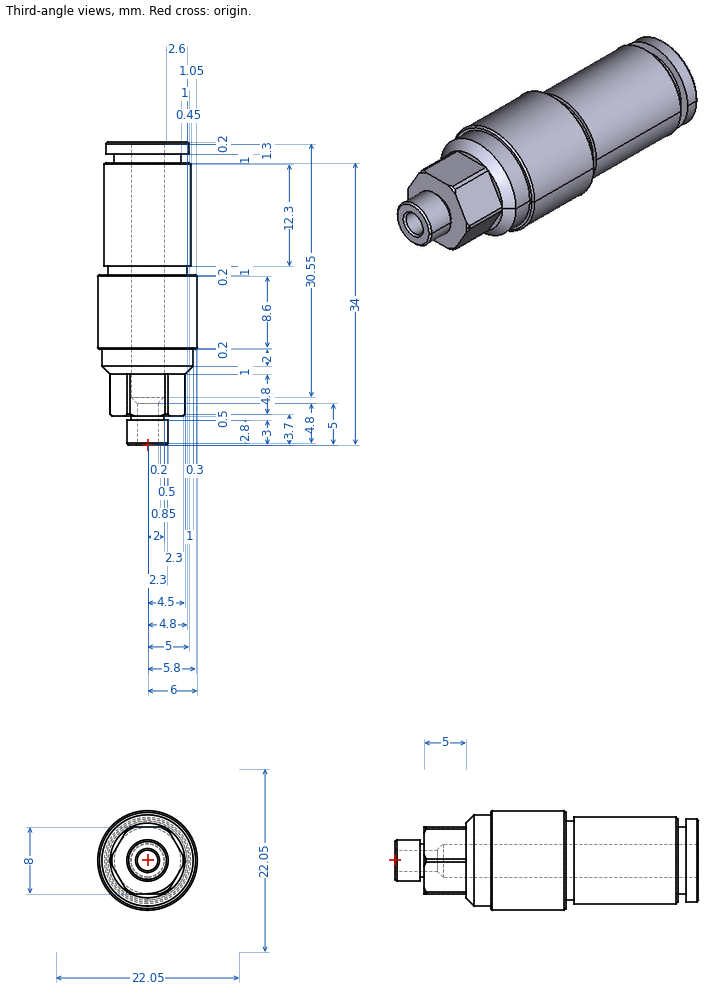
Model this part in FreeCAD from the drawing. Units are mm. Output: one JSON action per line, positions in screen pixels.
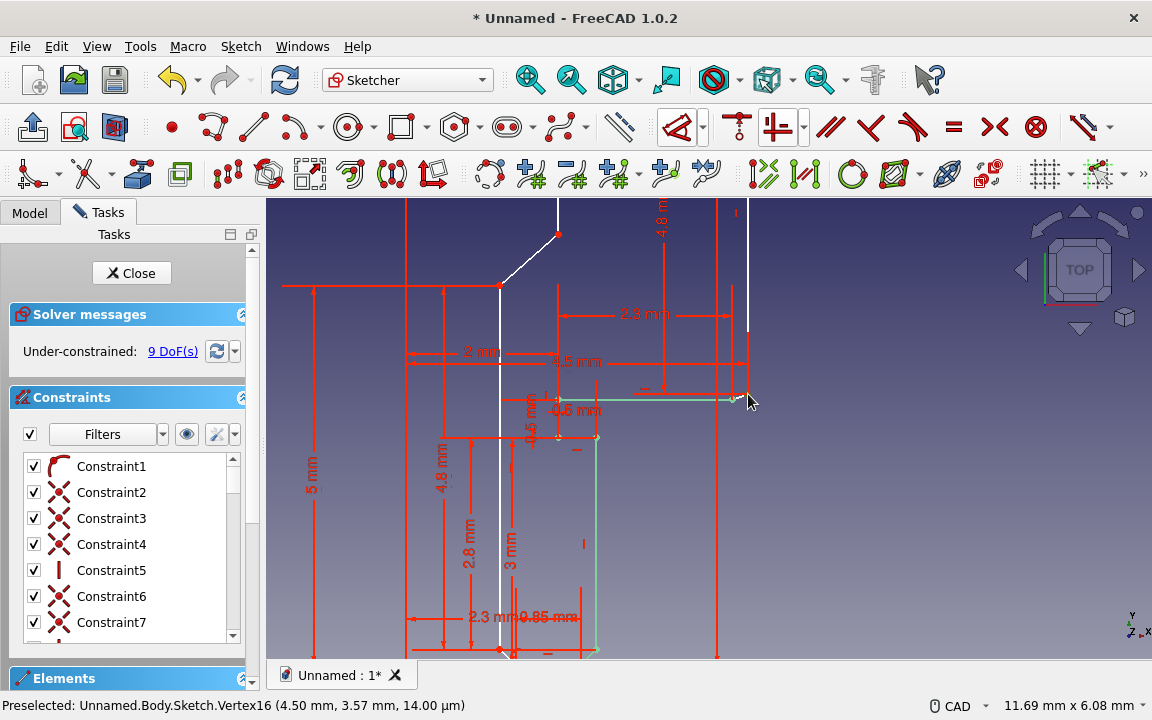
{"action": "key", "text": "i"}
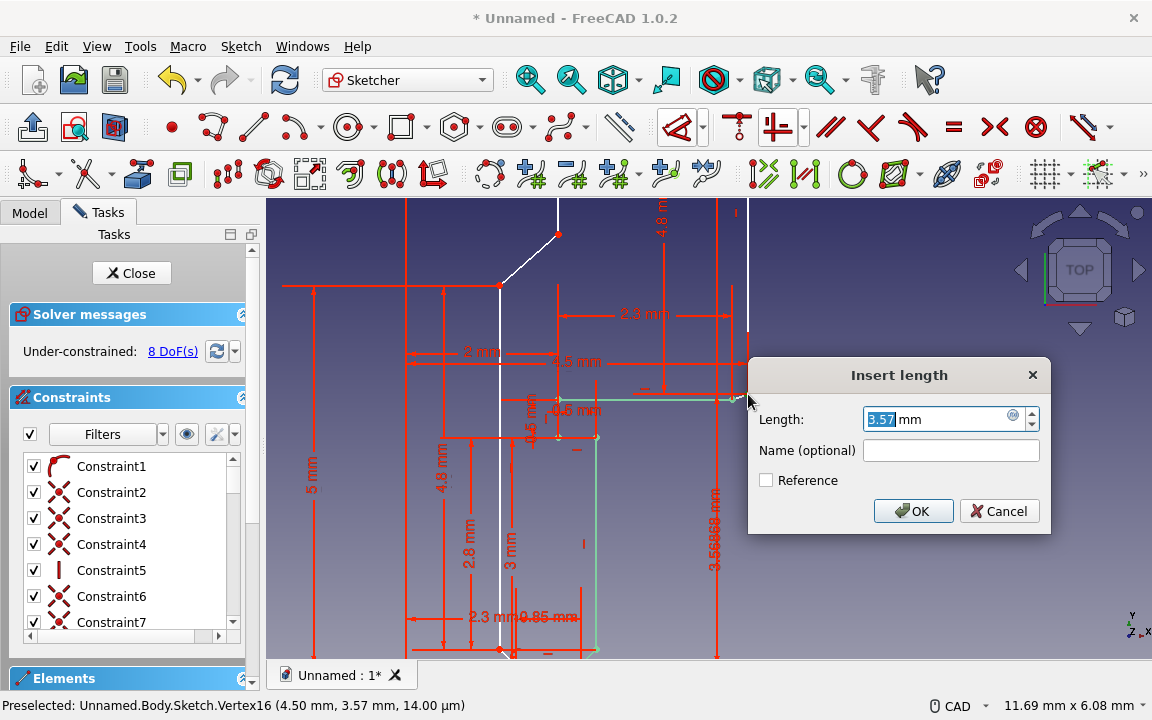
{"action": "type", "text": "3.7"}
{"action": "key", "text": "Return"}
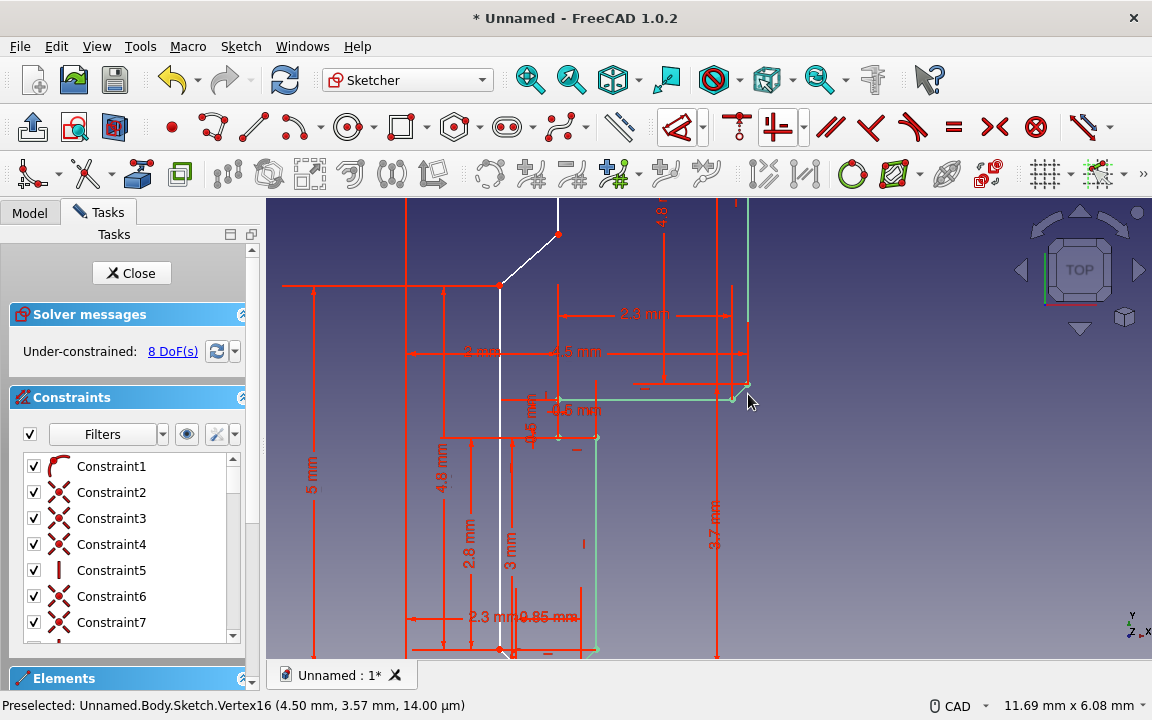
{"action": "scroll", "coordinate": [641, 571], "scroll_direction": "down", "scroll_amount": 11}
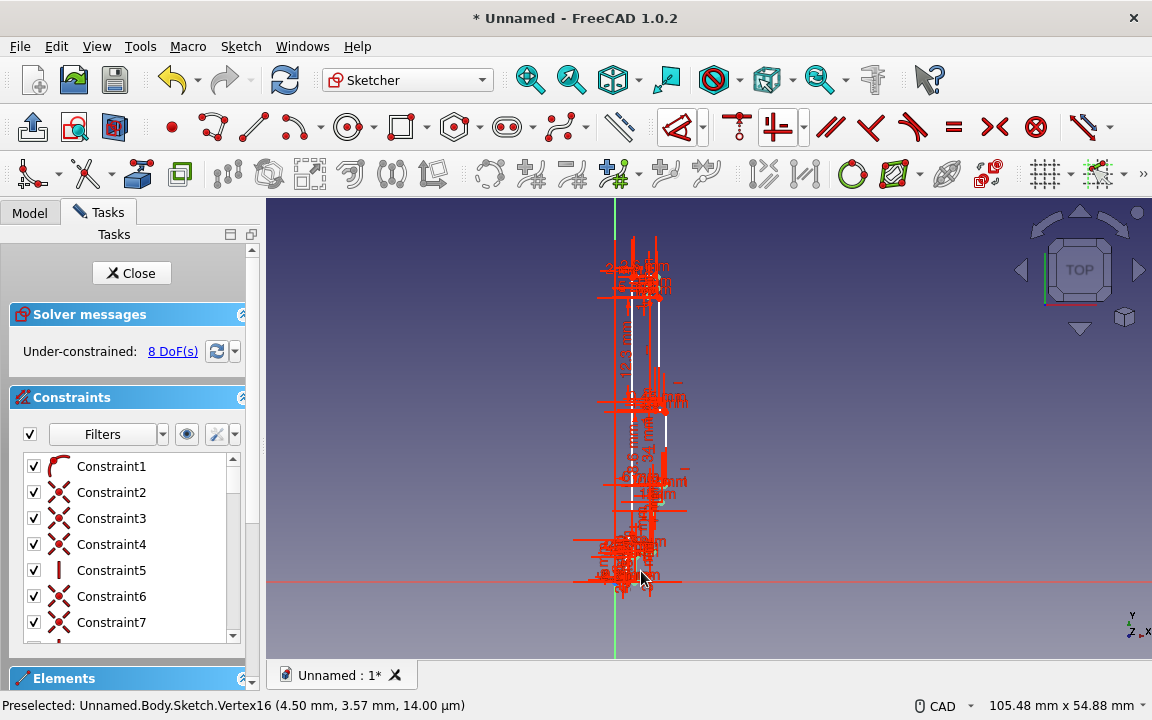
{"action": "scroll", "coordinate": [664, 410], "scroll_direction": "up", "scroll_amount": 8}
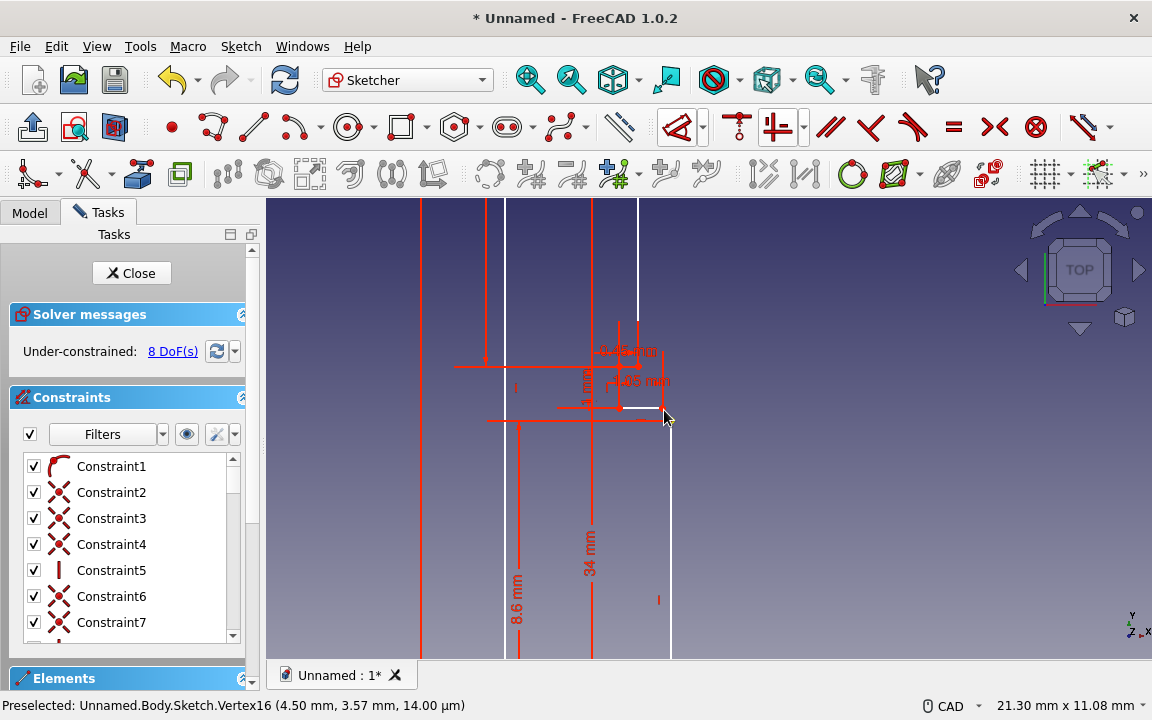
{"action": "left_click", "coordinate": [663, 408]}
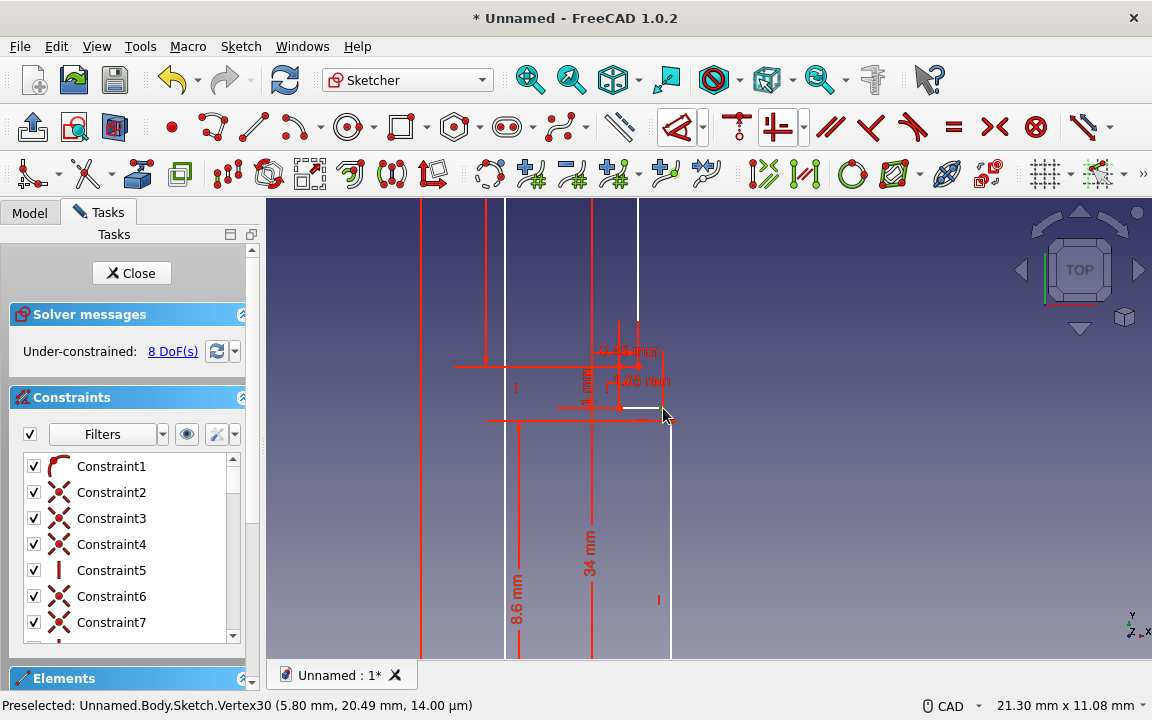
{"action": "left_click", "coordinate": [702, 128]}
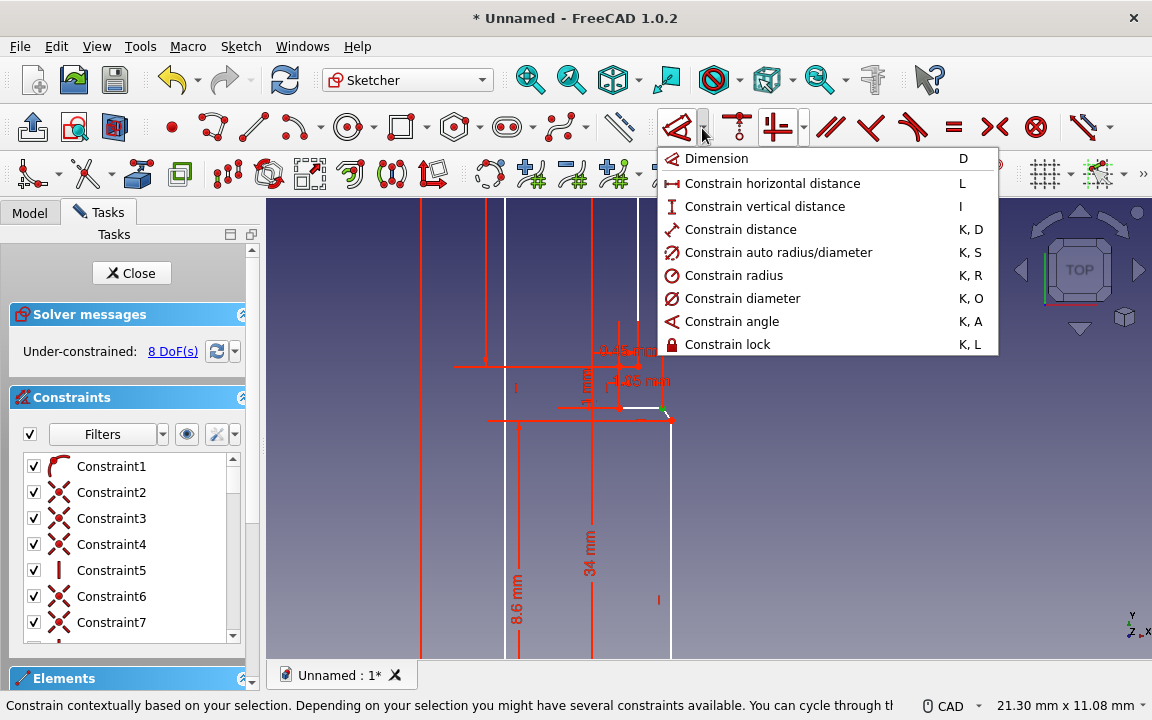
{"action": "left_click", "coordinate": [828, 184]}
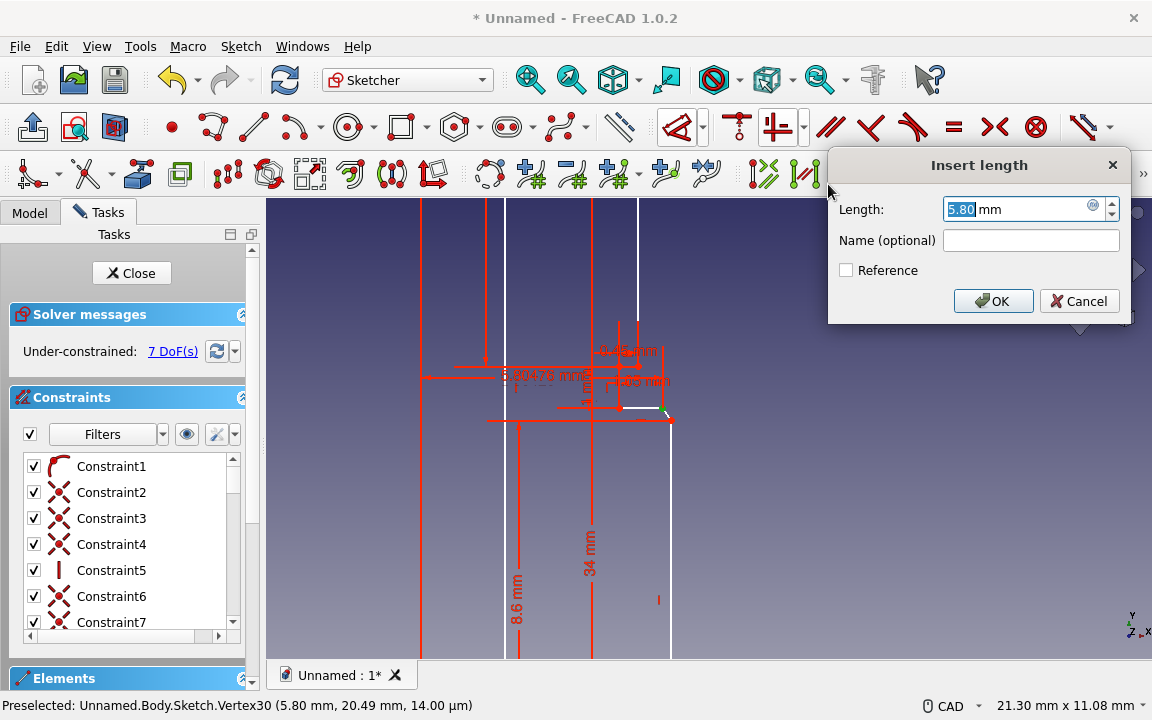
{"action": "type", "text": "5.8"}
{"action": "key", "text": "Return"}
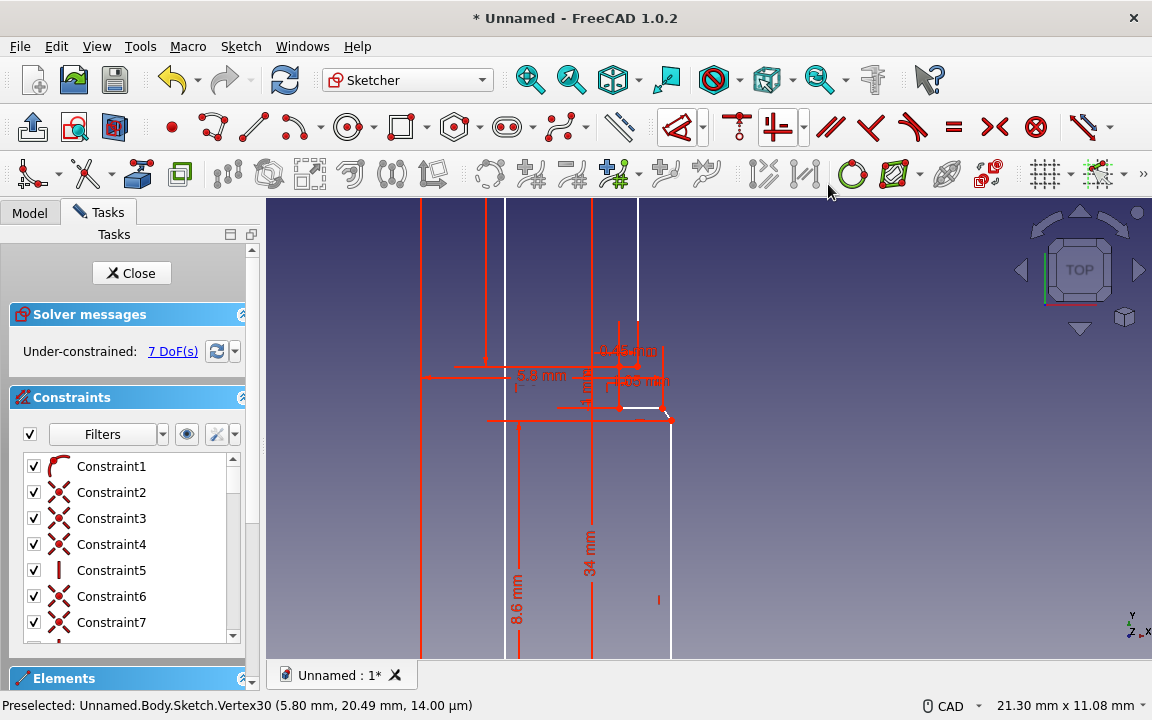
{"action": "scroll", "coordinate": [664, 410], "scroll_direction": "down", "scroll_amount": 8}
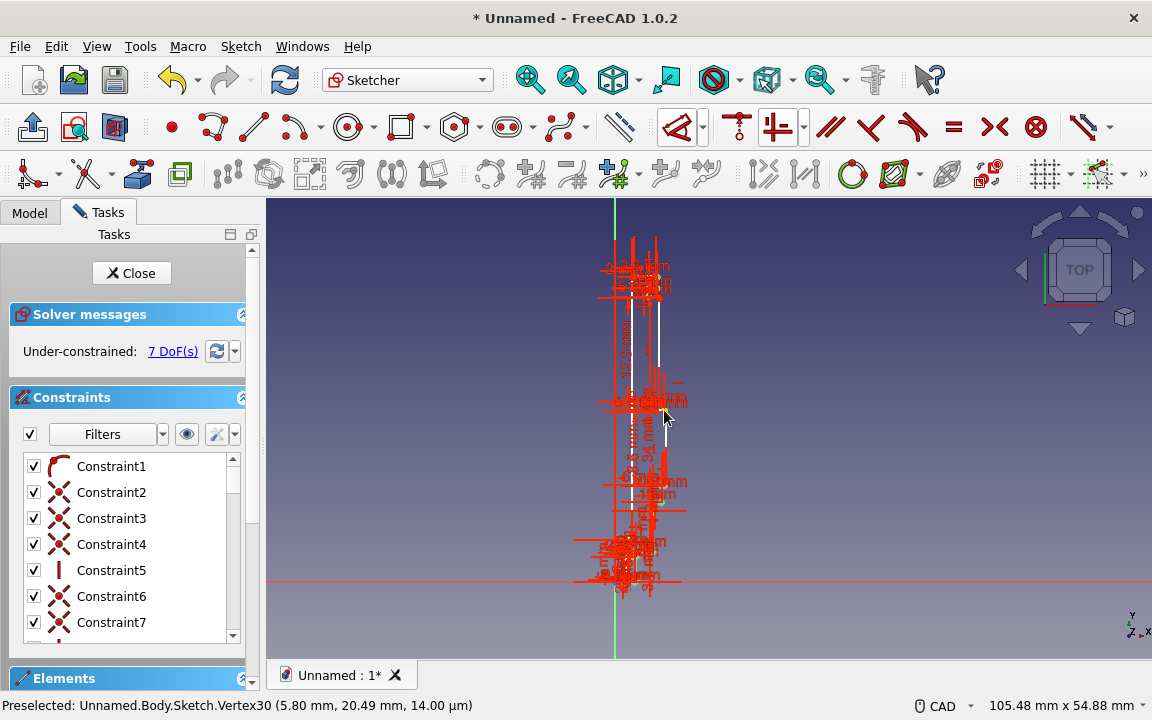
{"action": "scroll", "coordinate": [656, 276], "scroll_direction": "up", "scroll_amount": 9}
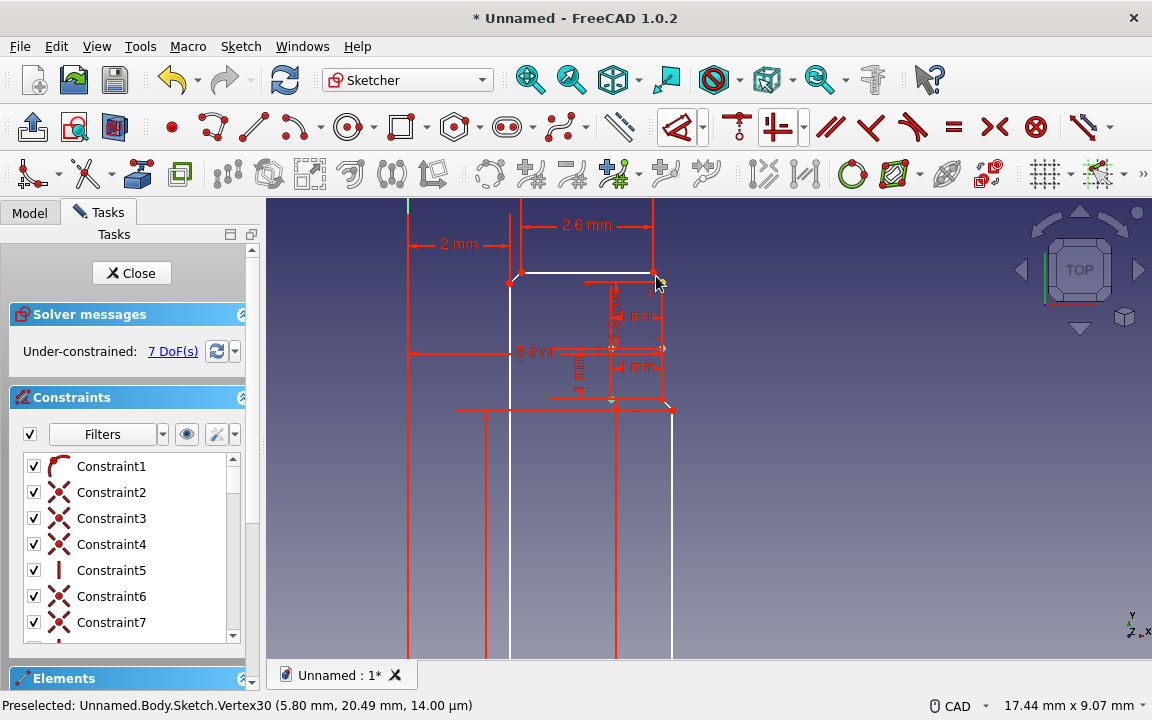
{"action": "left_click", "coordinate": [653, 273]}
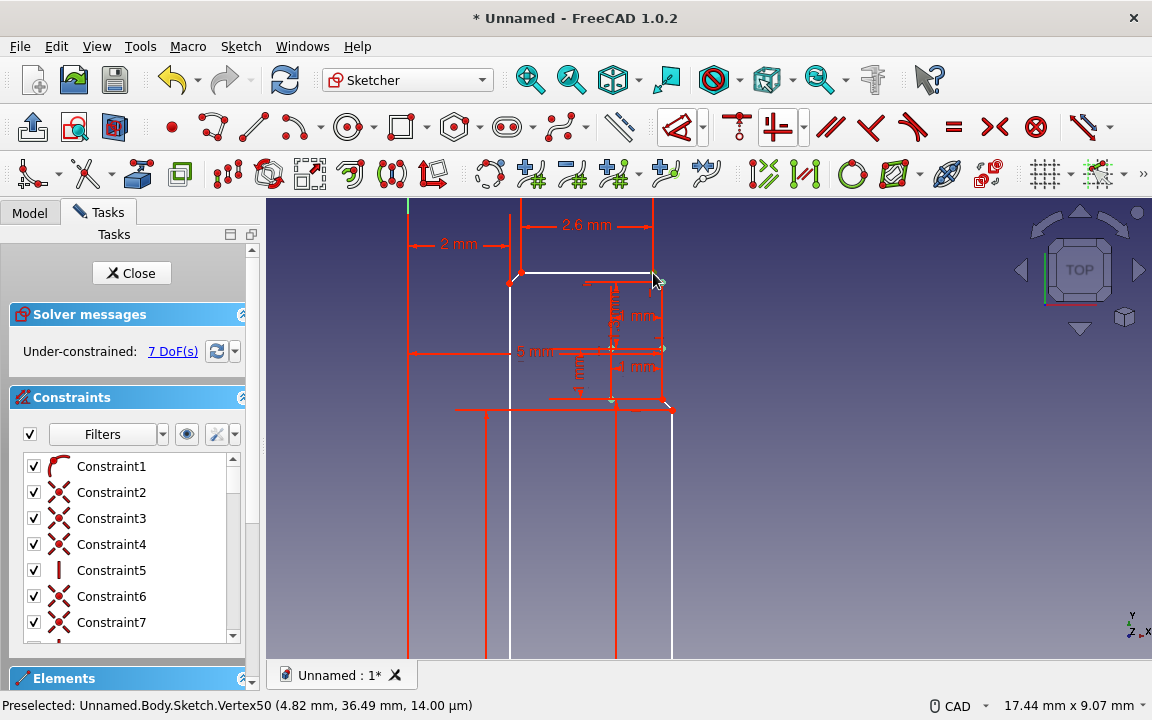
{"action": "left_click", "coordinate": [702, 128]}